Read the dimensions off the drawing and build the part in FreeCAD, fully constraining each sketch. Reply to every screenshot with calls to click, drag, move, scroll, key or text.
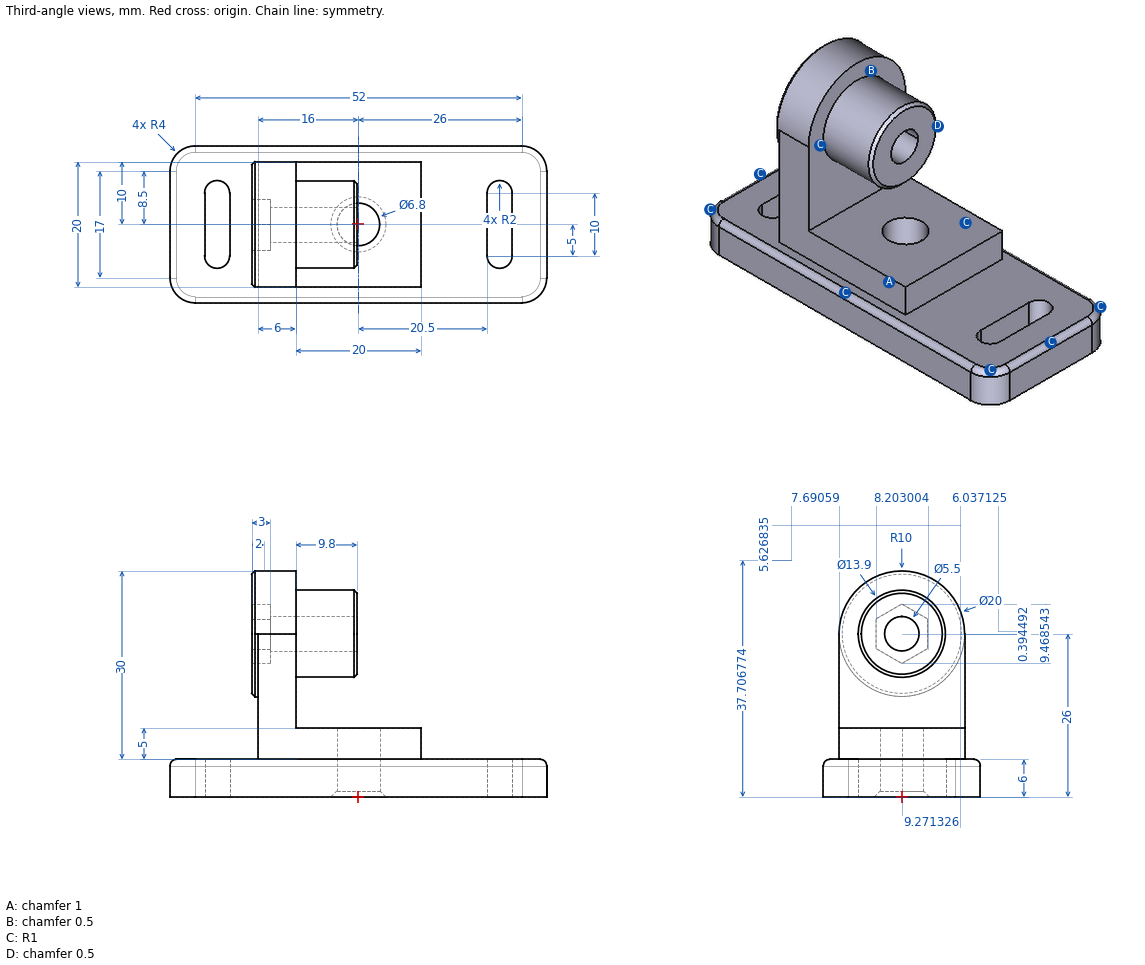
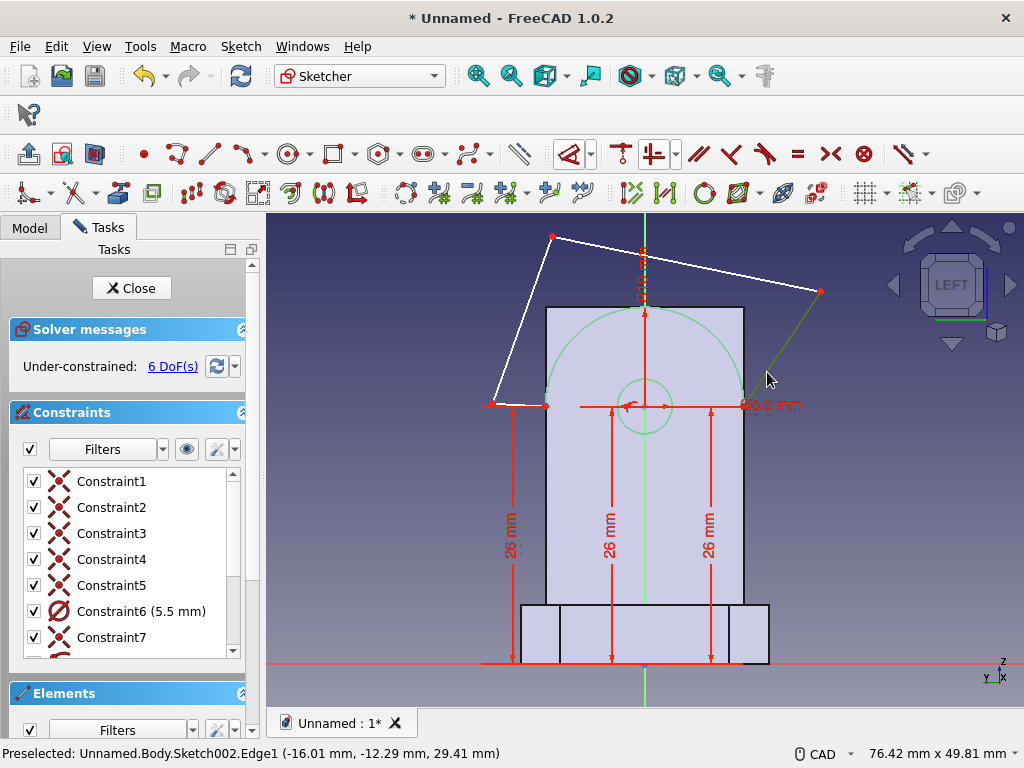
key(l)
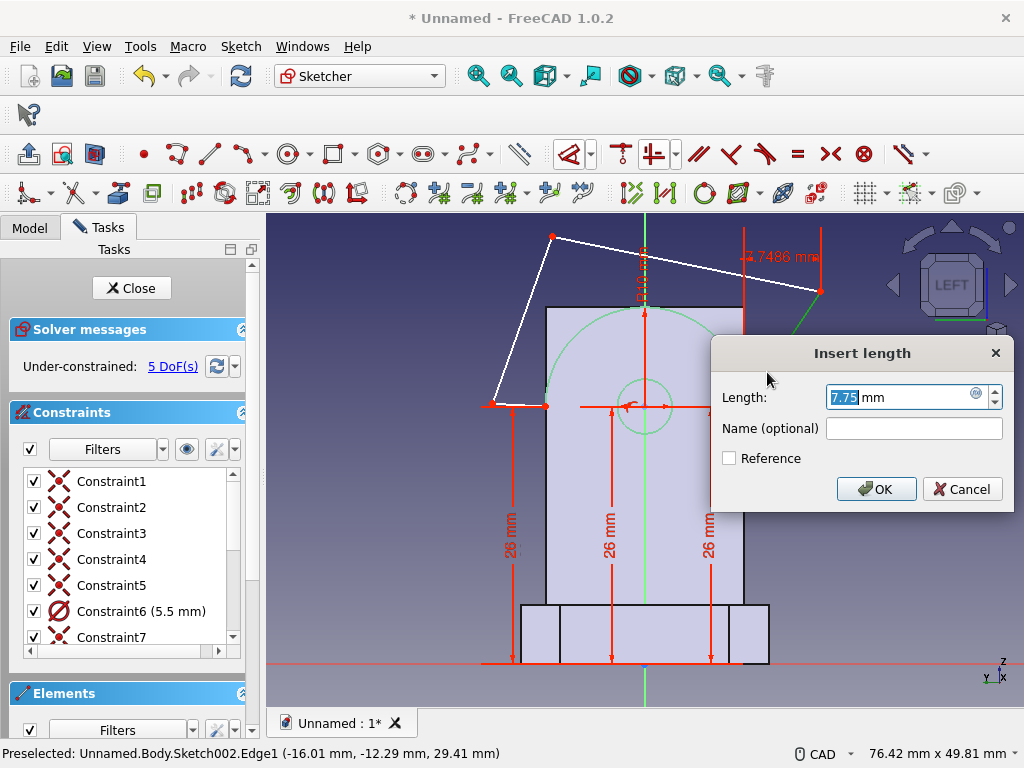
text(7.69059)
key(Return)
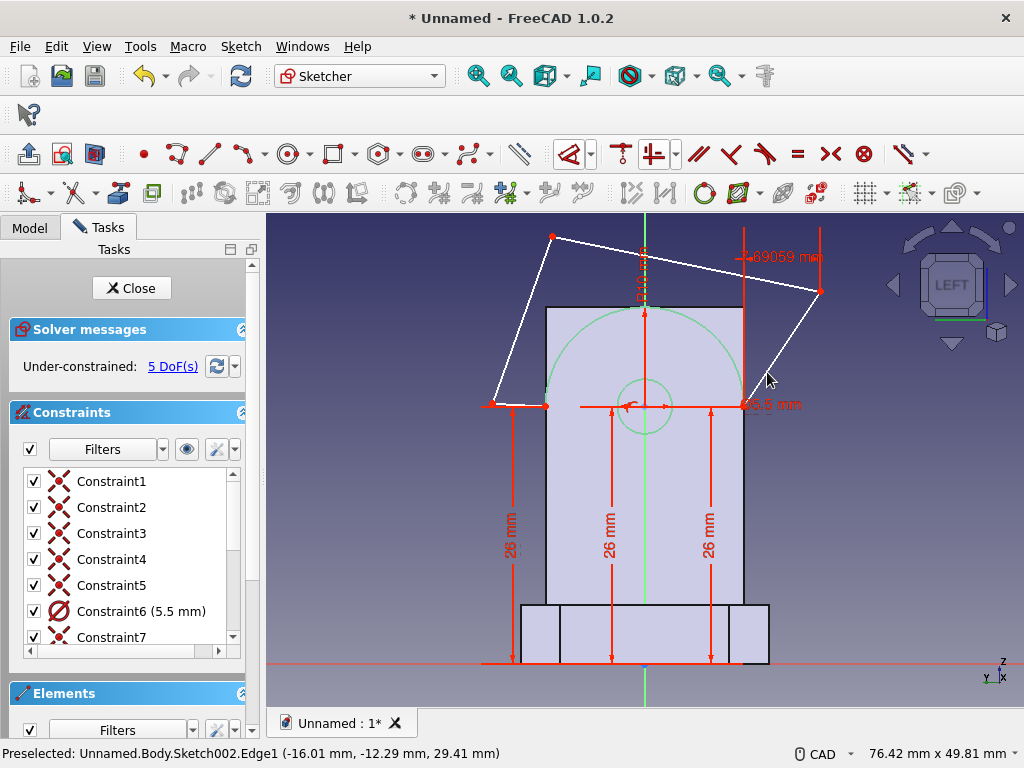
scroll(414, 481, down, 2)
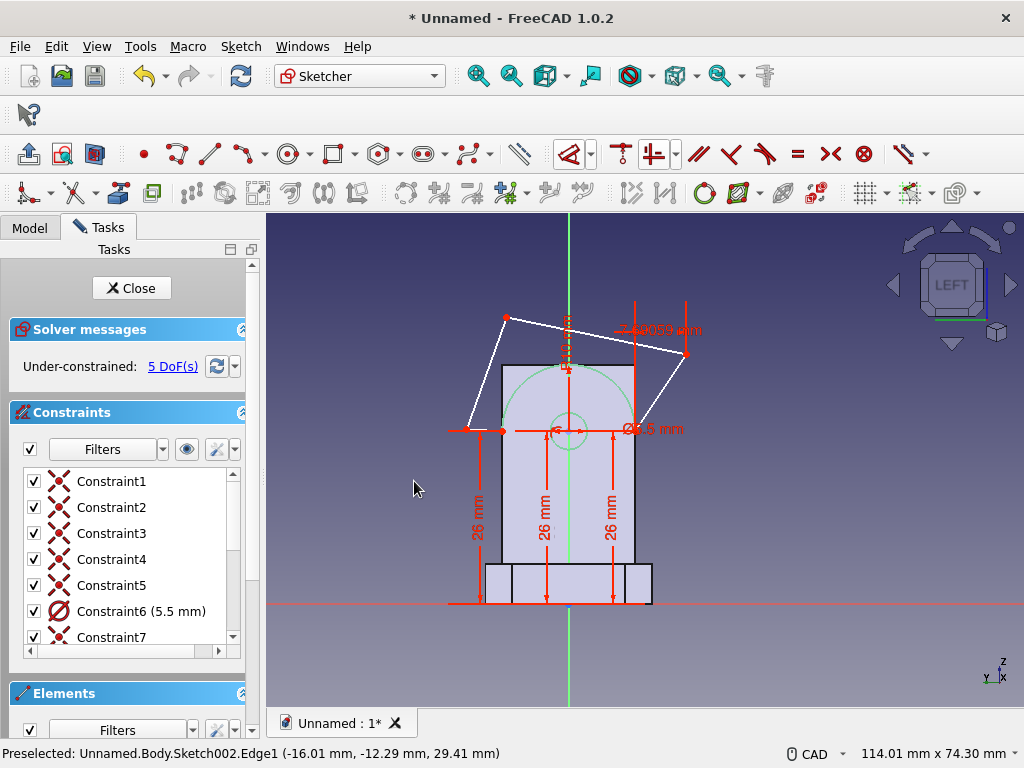
click(507, 317)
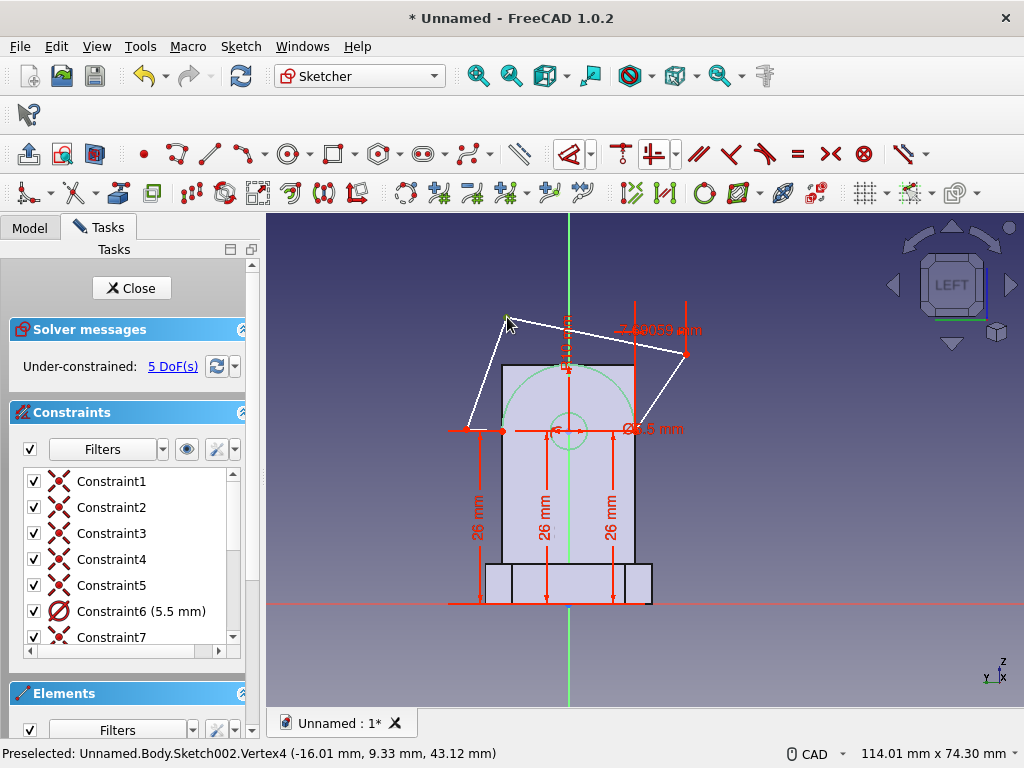
click(590, 154)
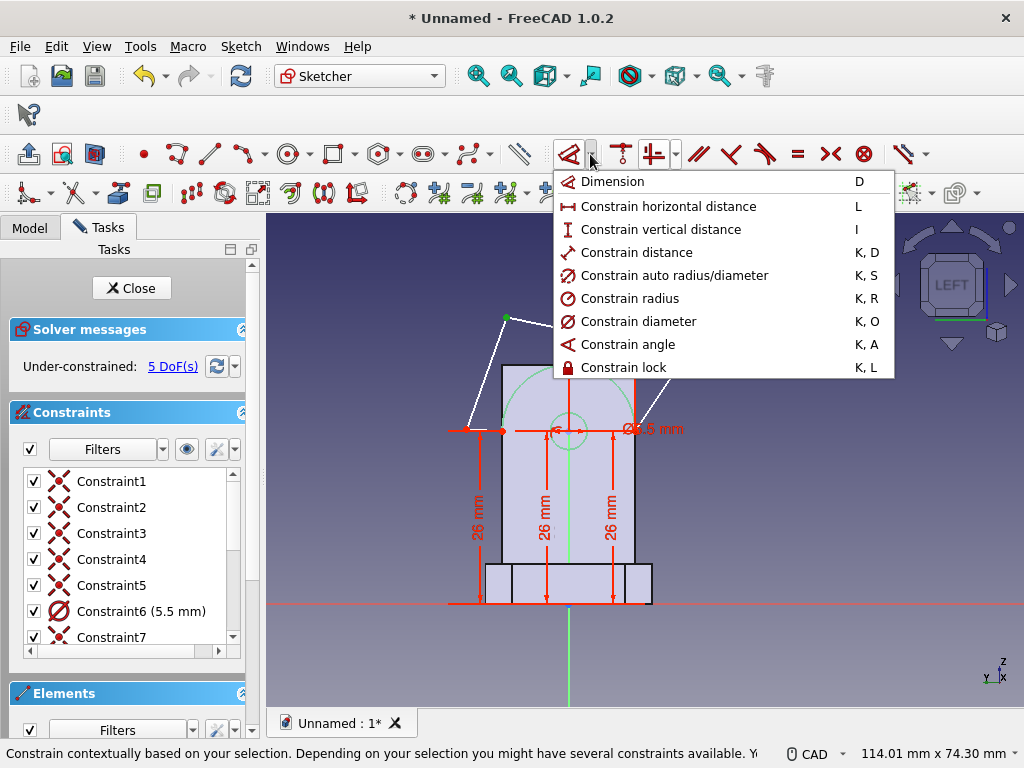
click(724, 206)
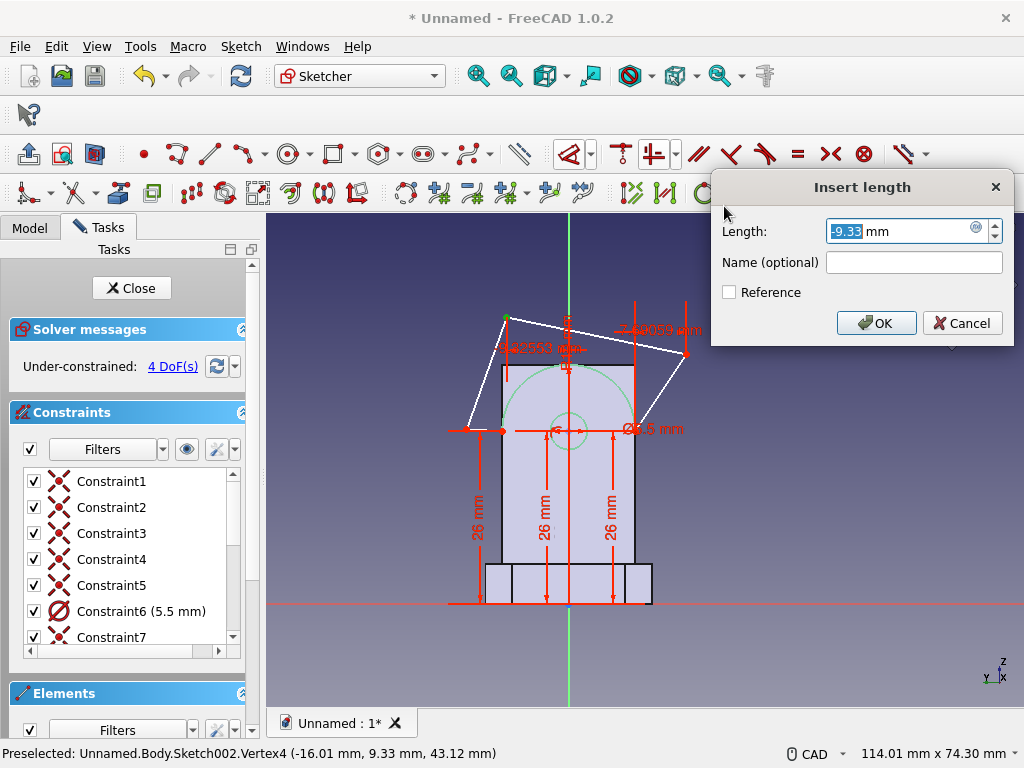
text(-9.271326)
key(Return)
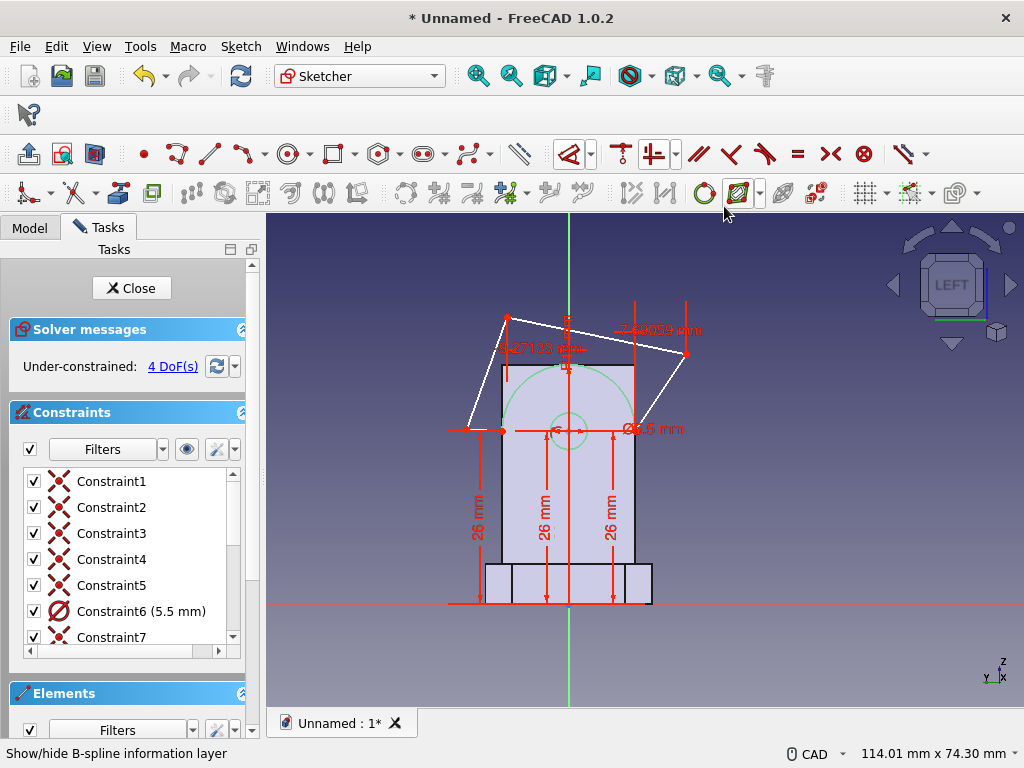
click(633, 343)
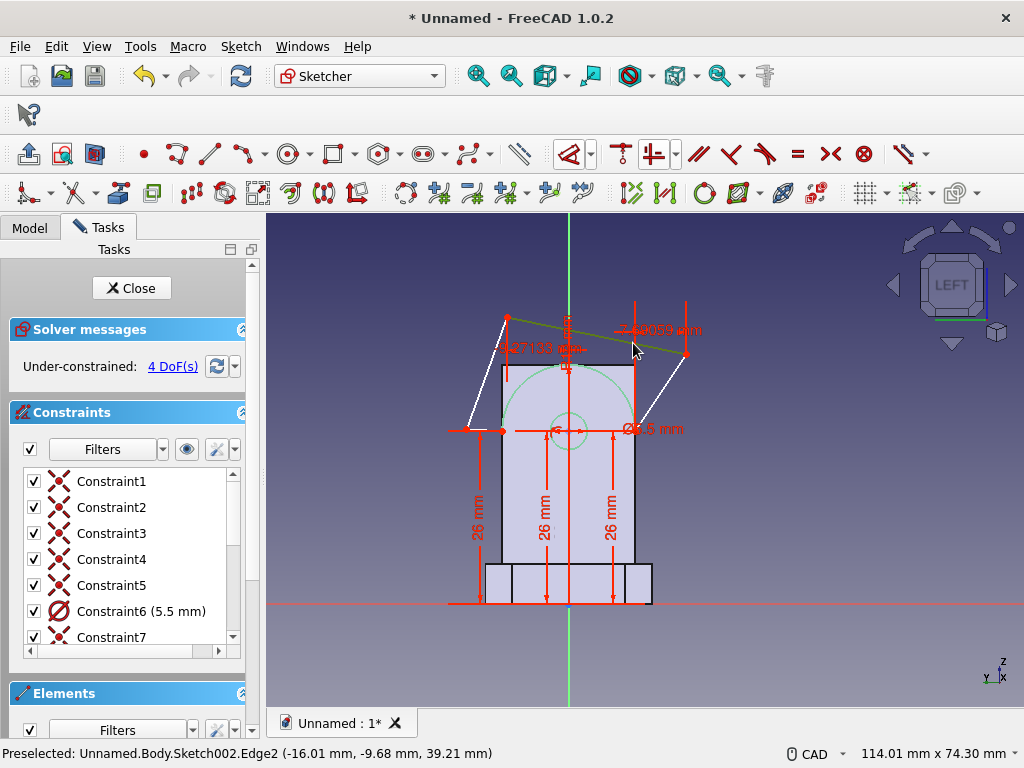
key(i)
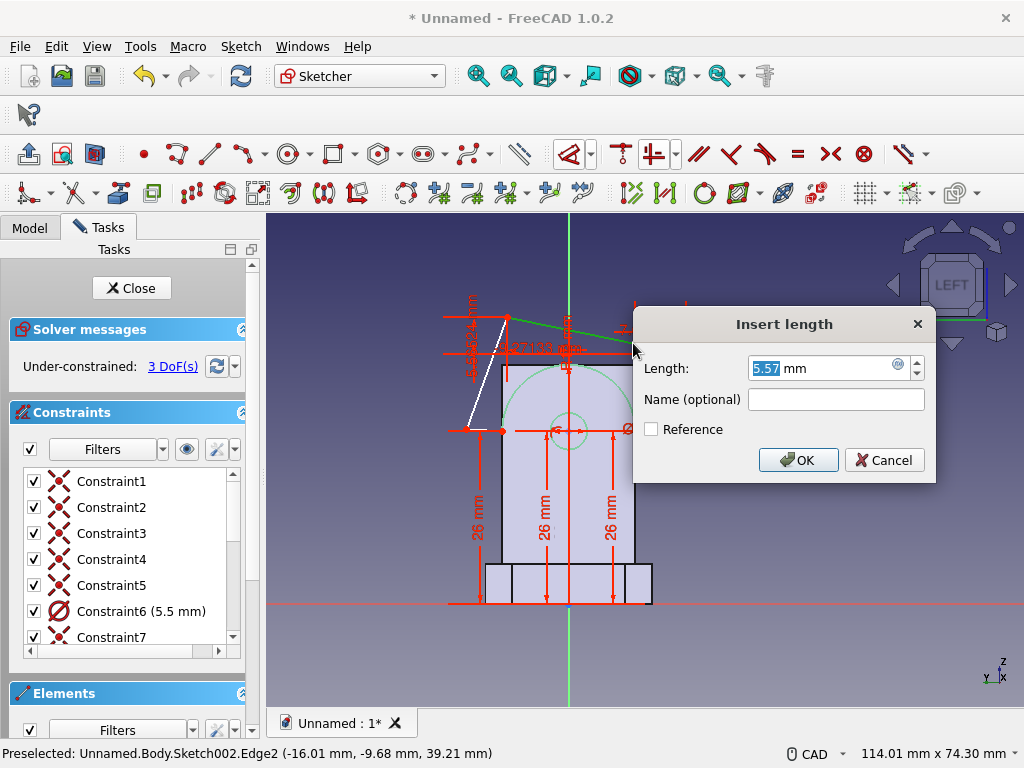
text(5.626835)
key(Return)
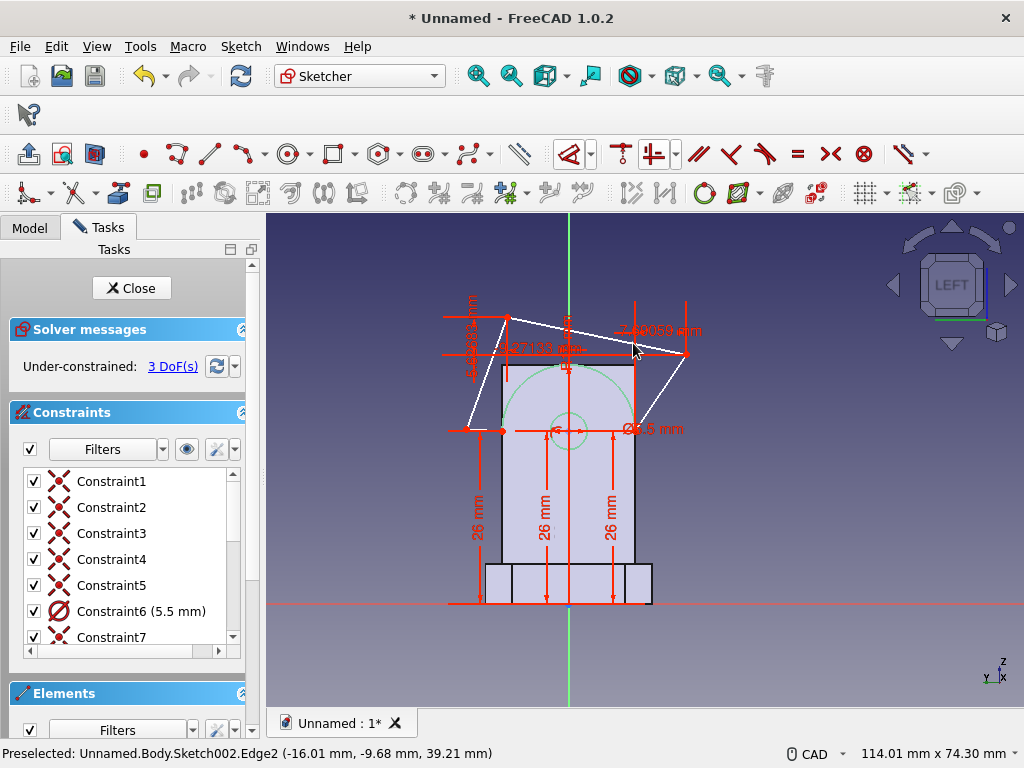
click(479, 396)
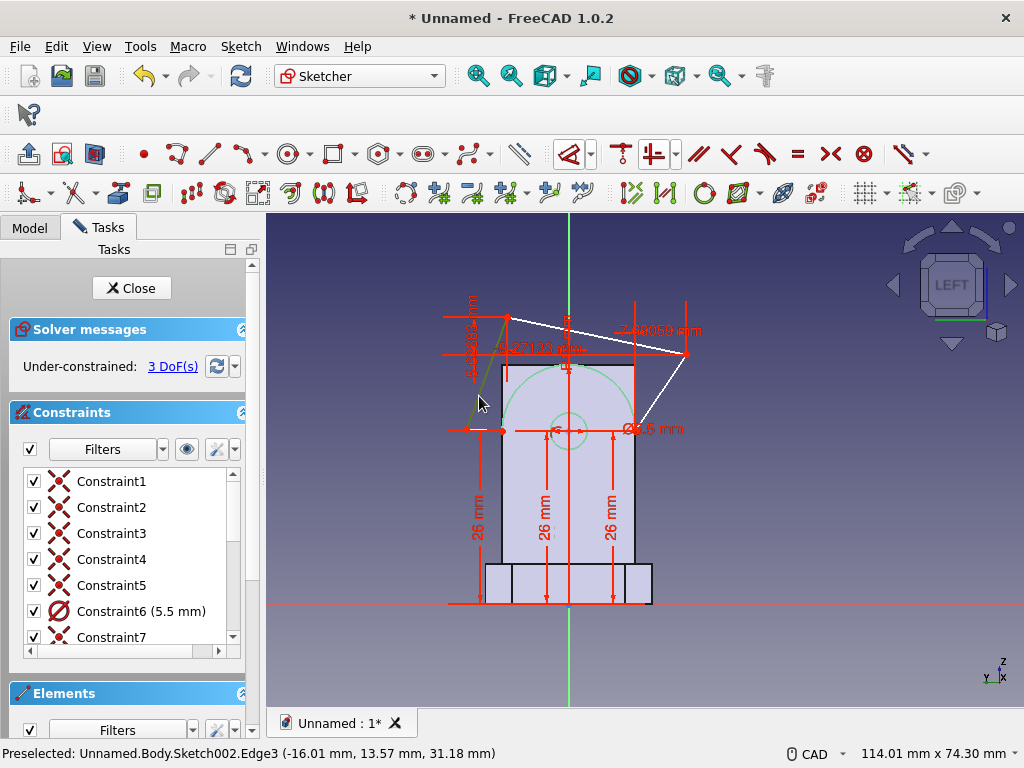
click(590, 154)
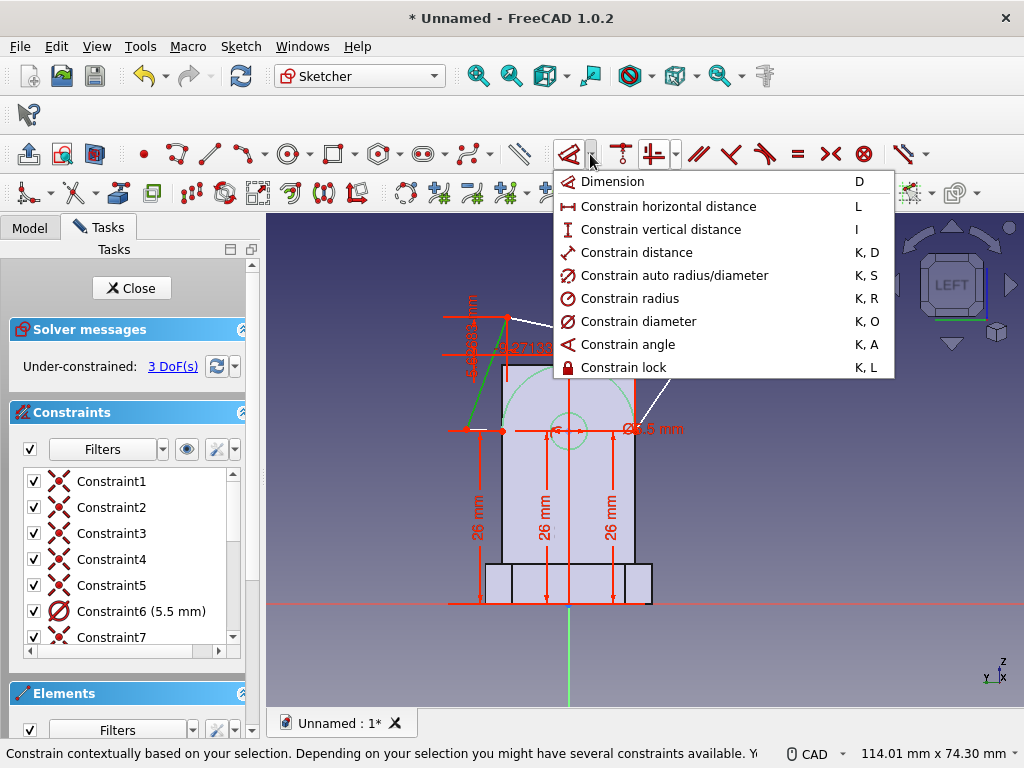
click(724, 206)